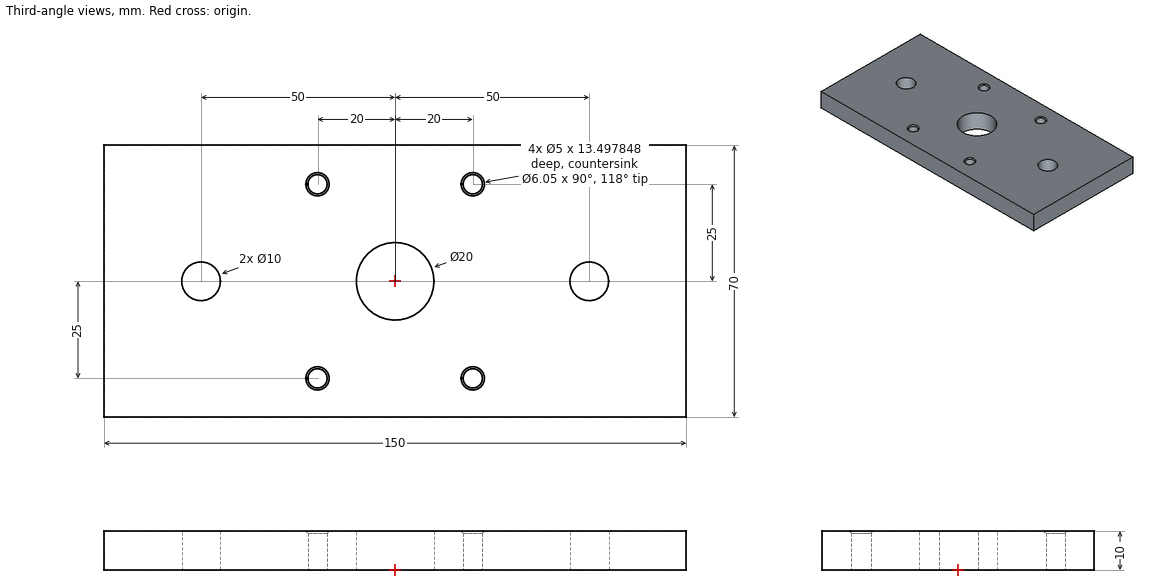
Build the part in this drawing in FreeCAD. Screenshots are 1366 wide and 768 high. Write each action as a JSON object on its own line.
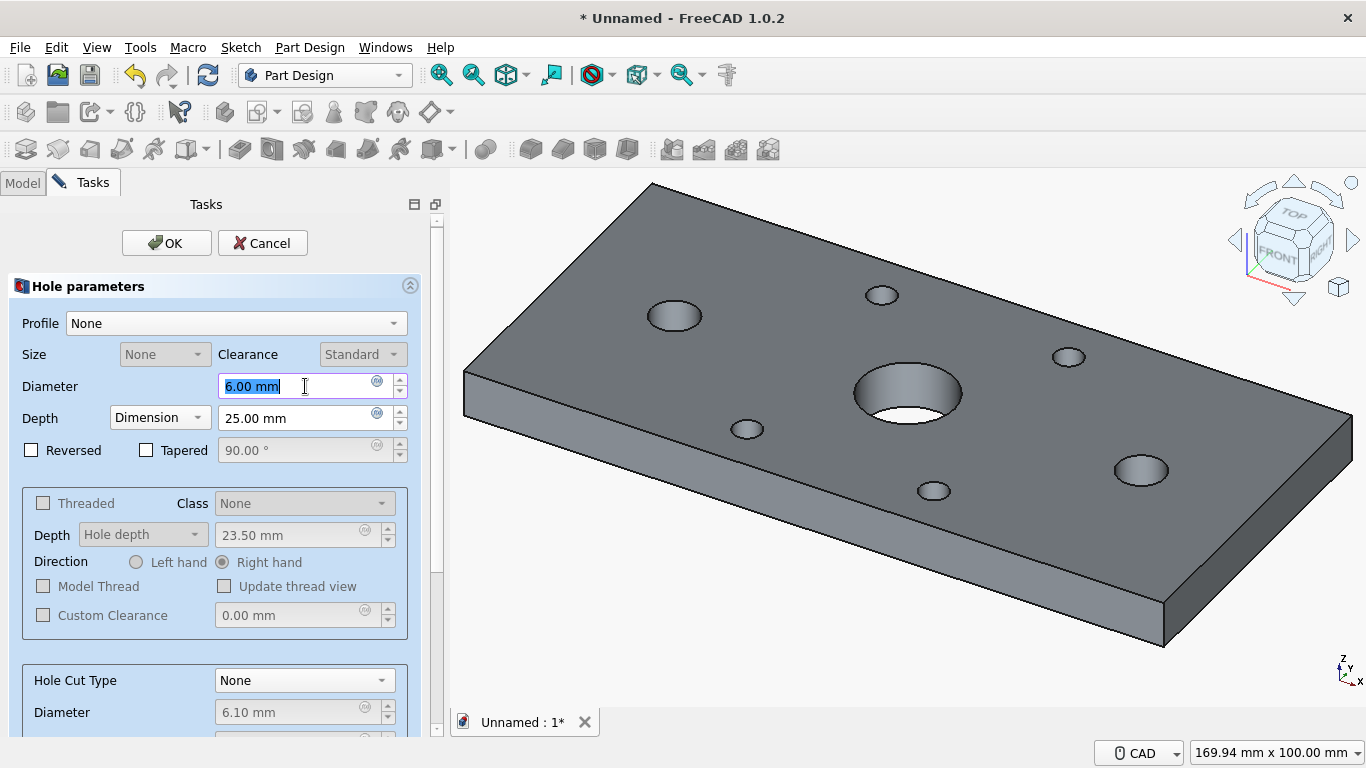
{"action": "type", "text": "5"}
{"action": "key", "text": "Tab"}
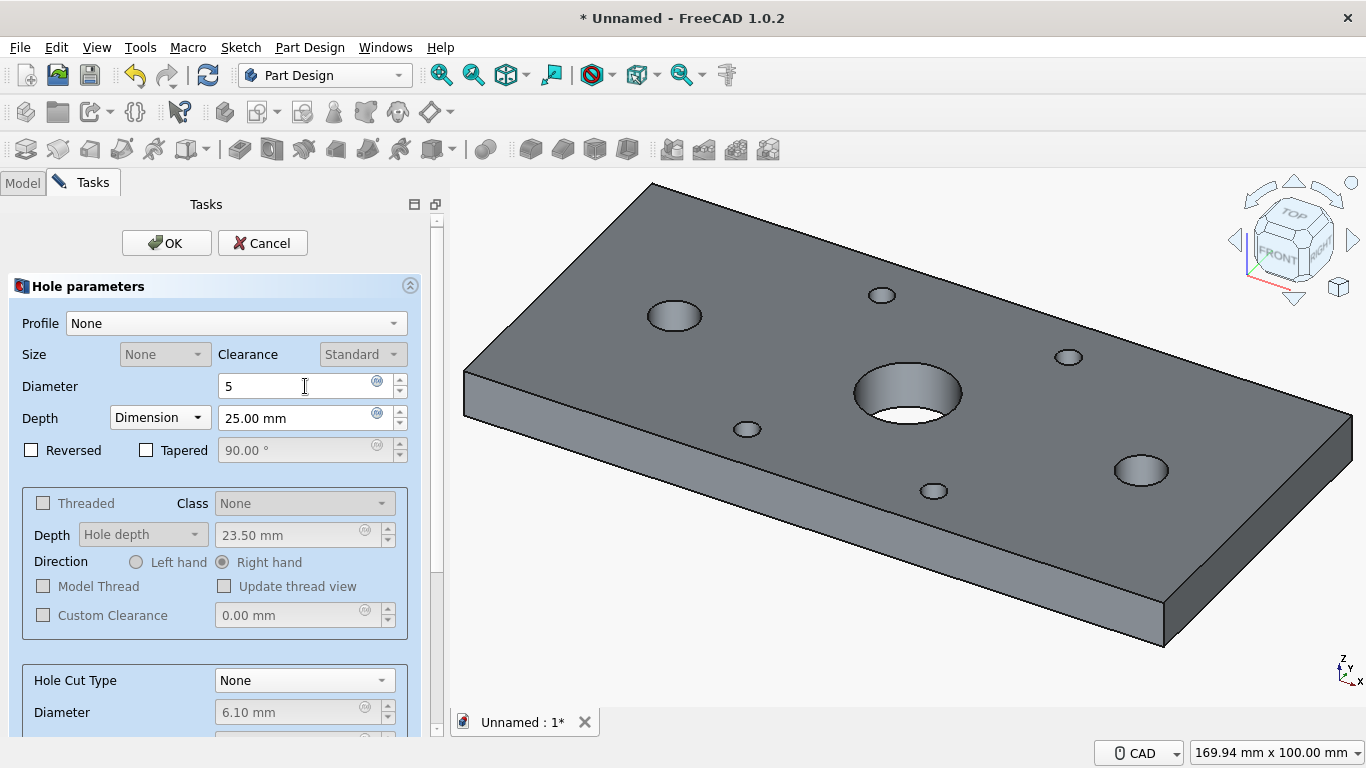
{"action": "triple_click", "coordinate": [305, 418]}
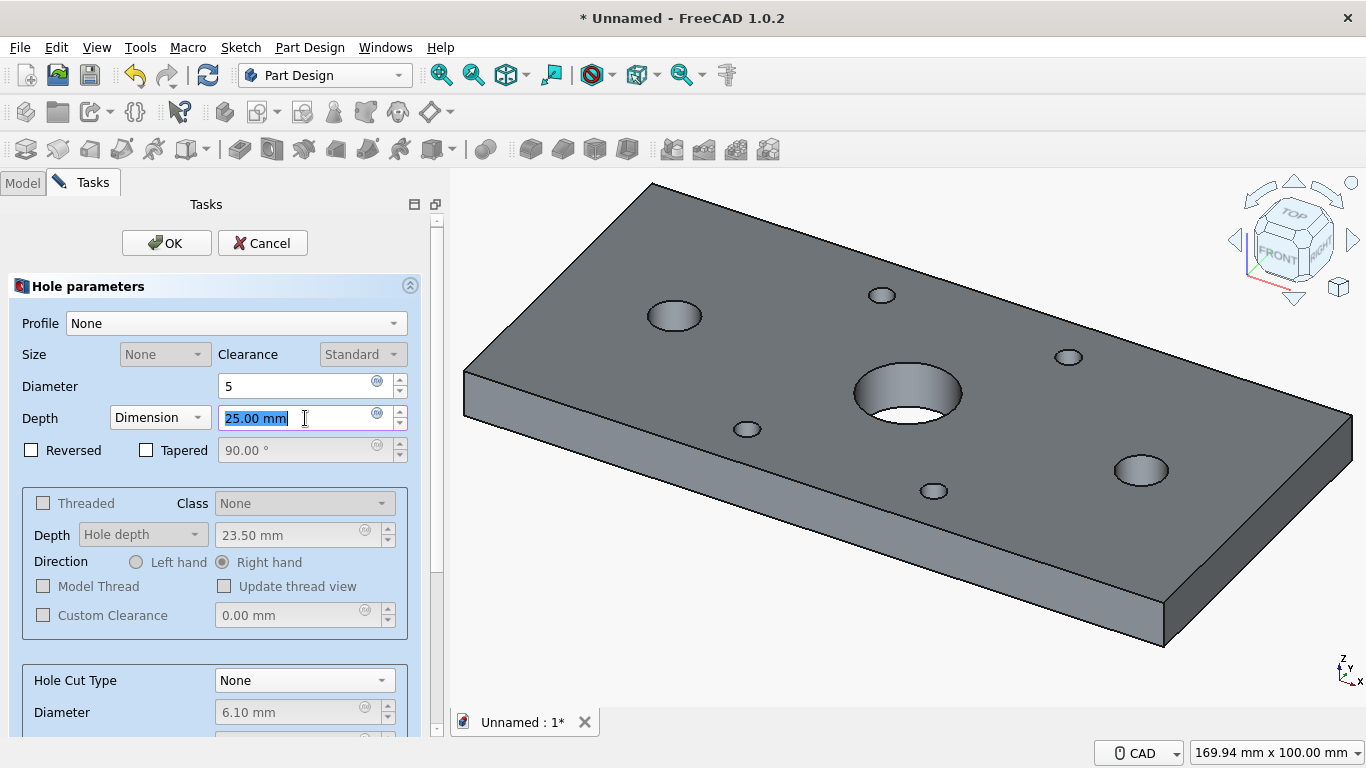
{"action": "type", "text": "13.497848"}
{"action": "key", "text": "Tab"}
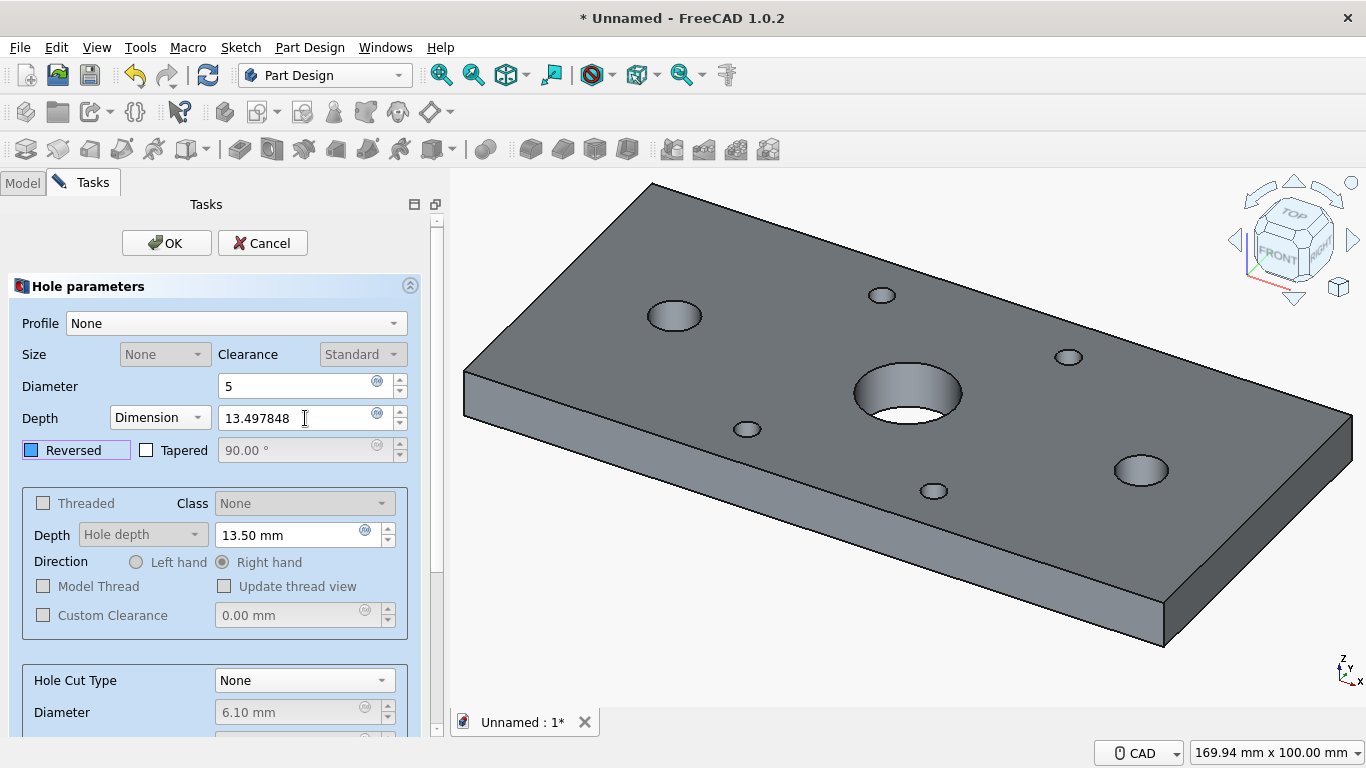
{"action": "left_click", "coordinate": [306, 680]}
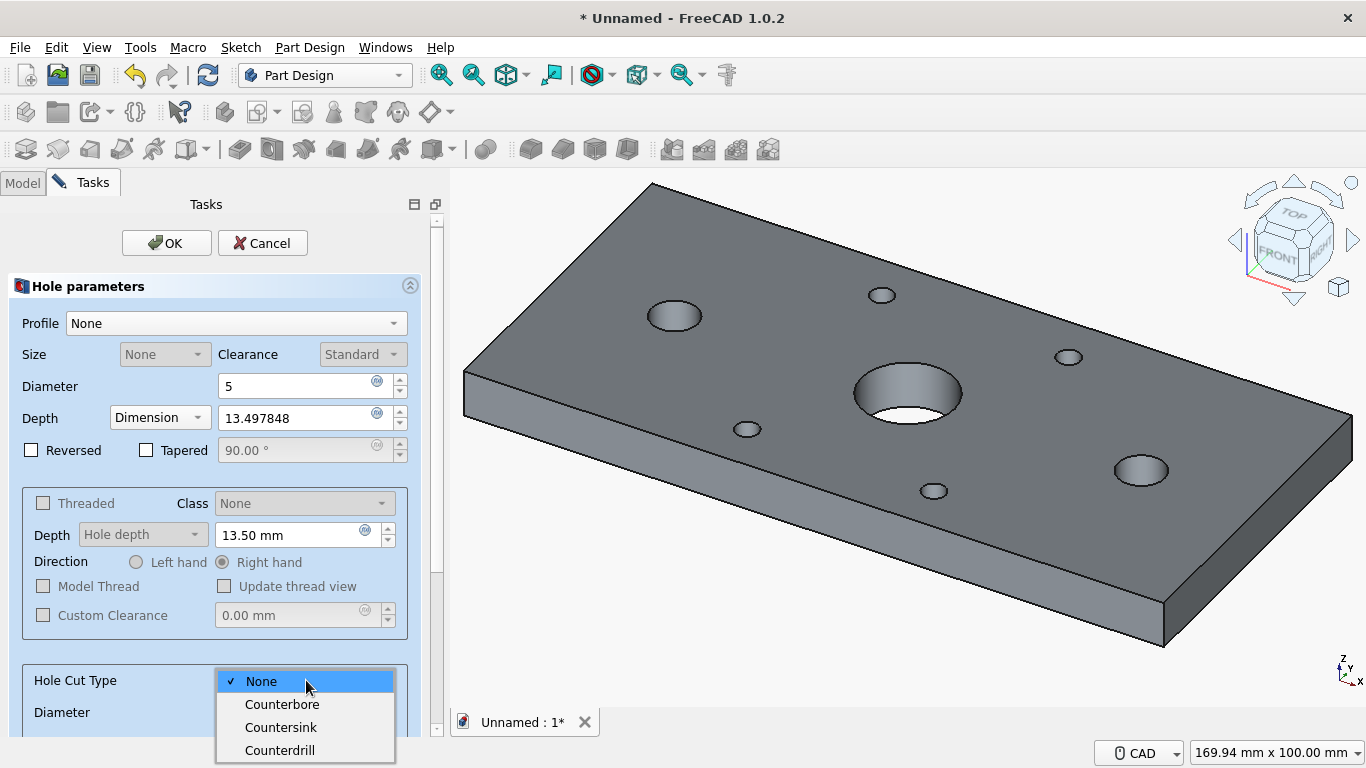
{"action": "left_click", "coordinate": [304, 728]}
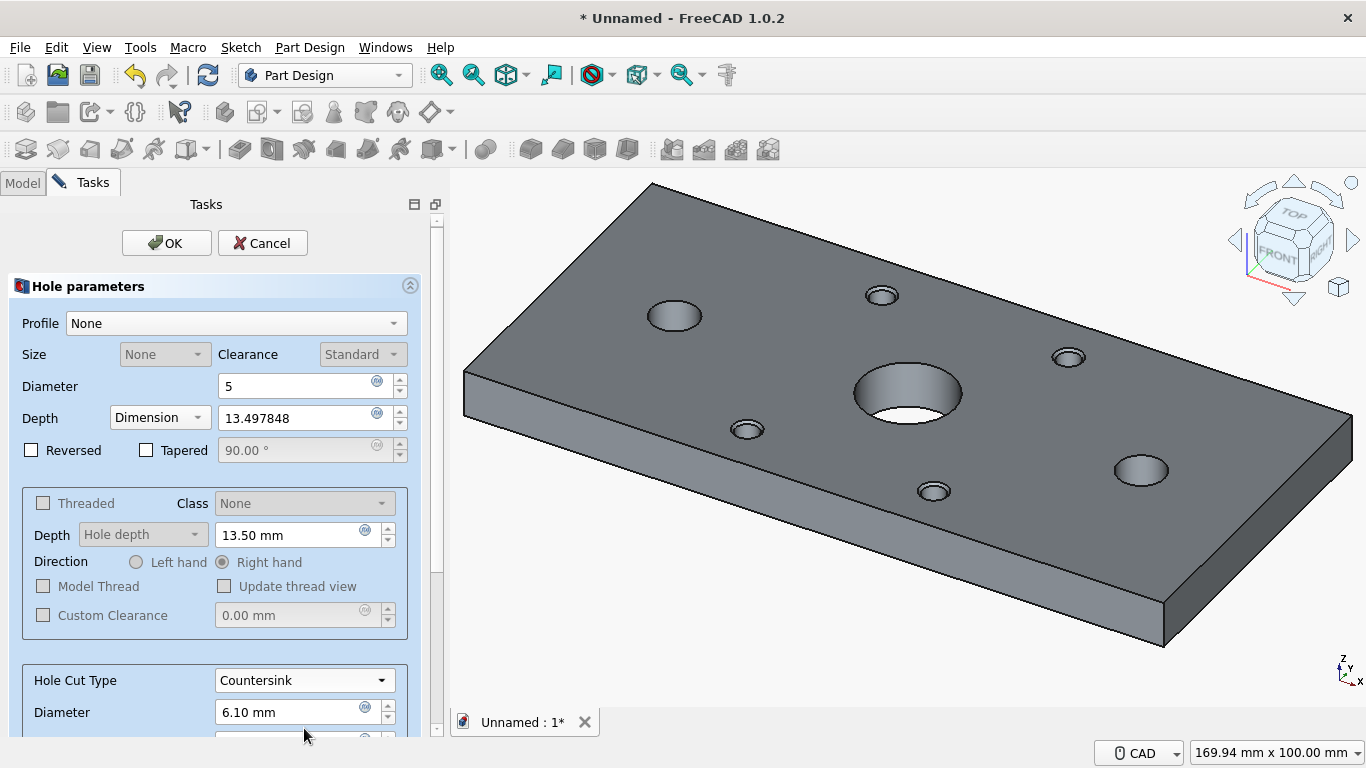
{"action": "triple_click", "coordinate": [298, 712]}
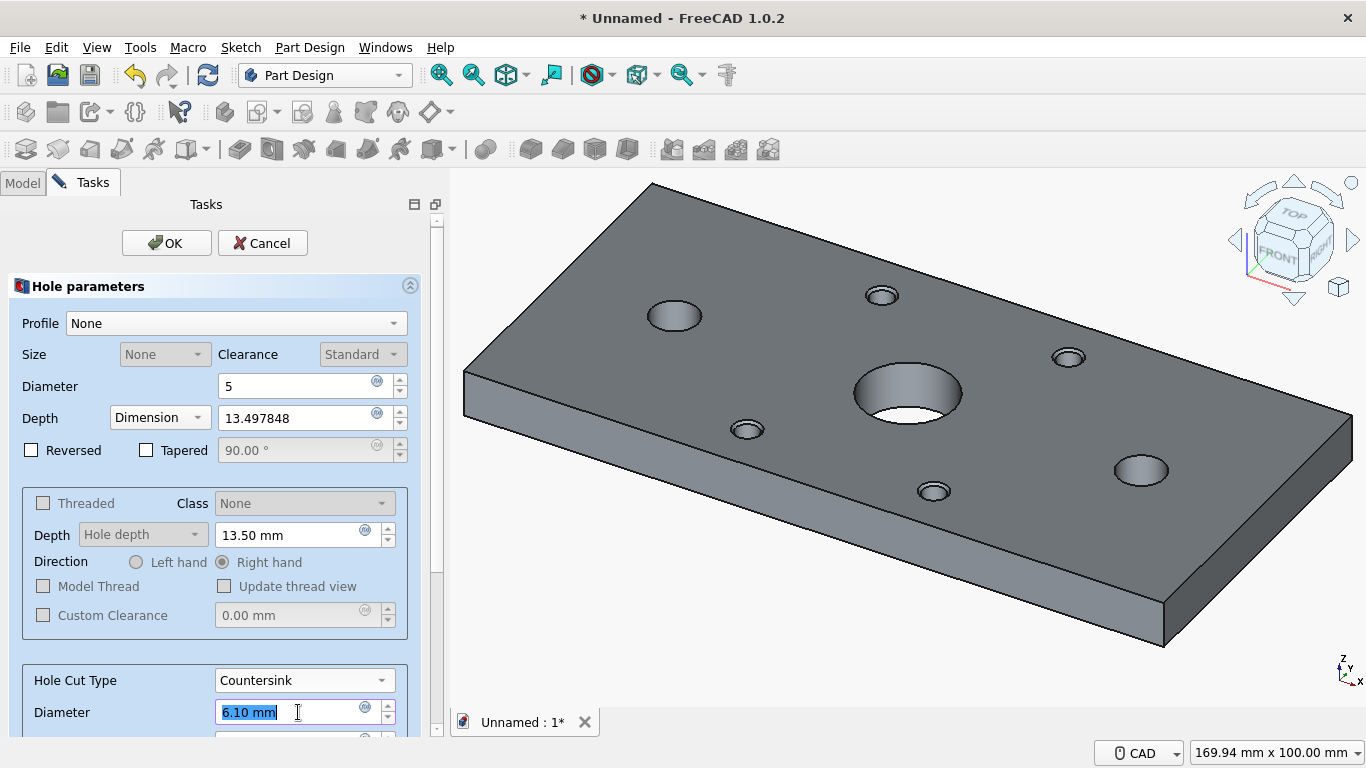
{"action": "type", "text": "6.05"}
{"action": "key", "text": "Tab"}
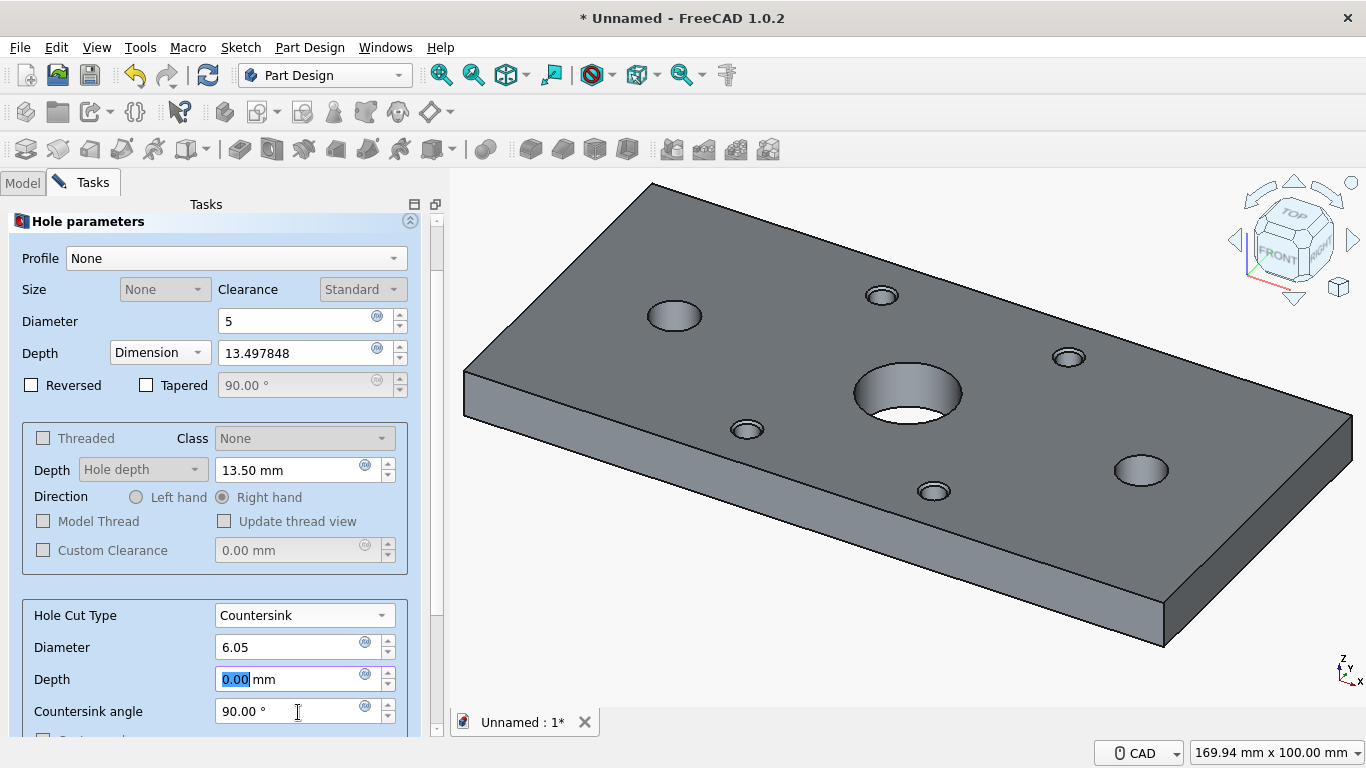
{"action": "scroll", "coordinate": [437, 475], "scroll_direction": "up", "scroll_amount": 2}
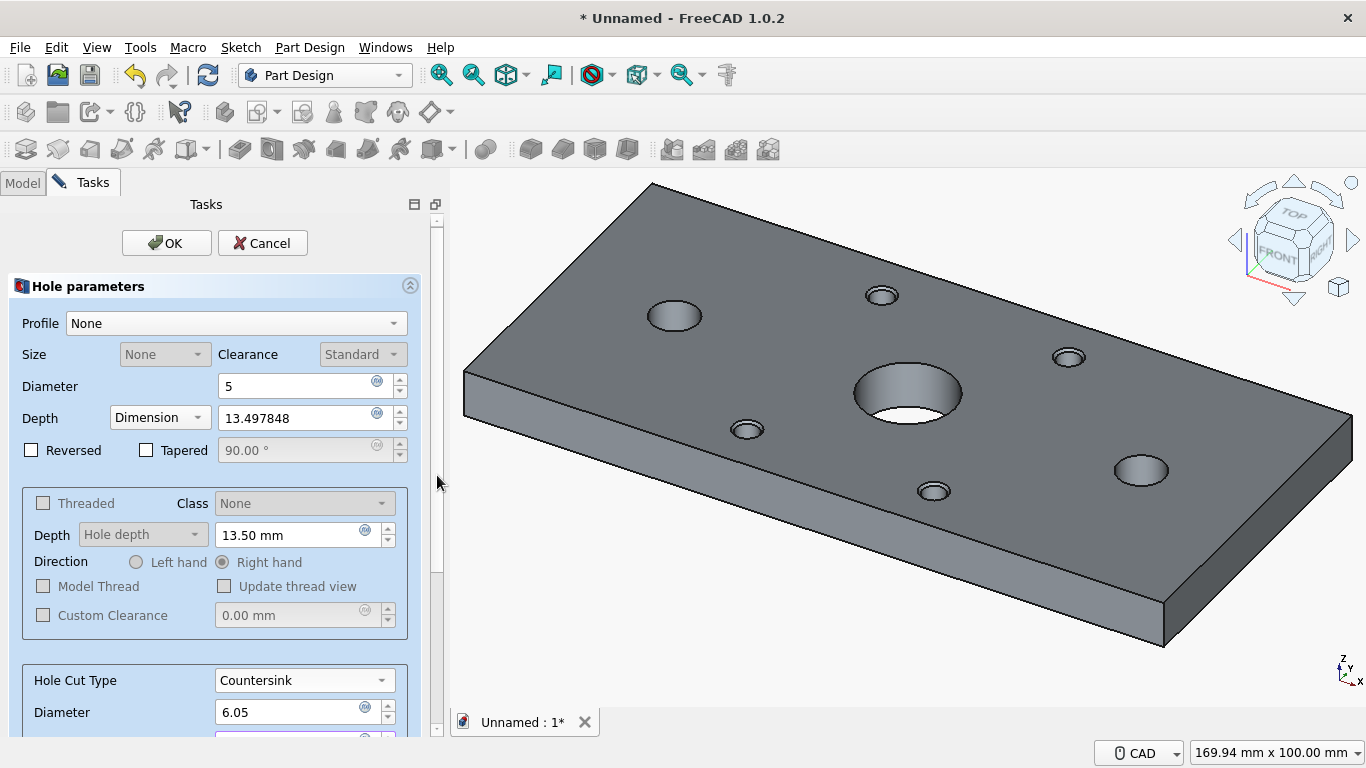
{"action": "left_click", "coordinate": [167, 243]}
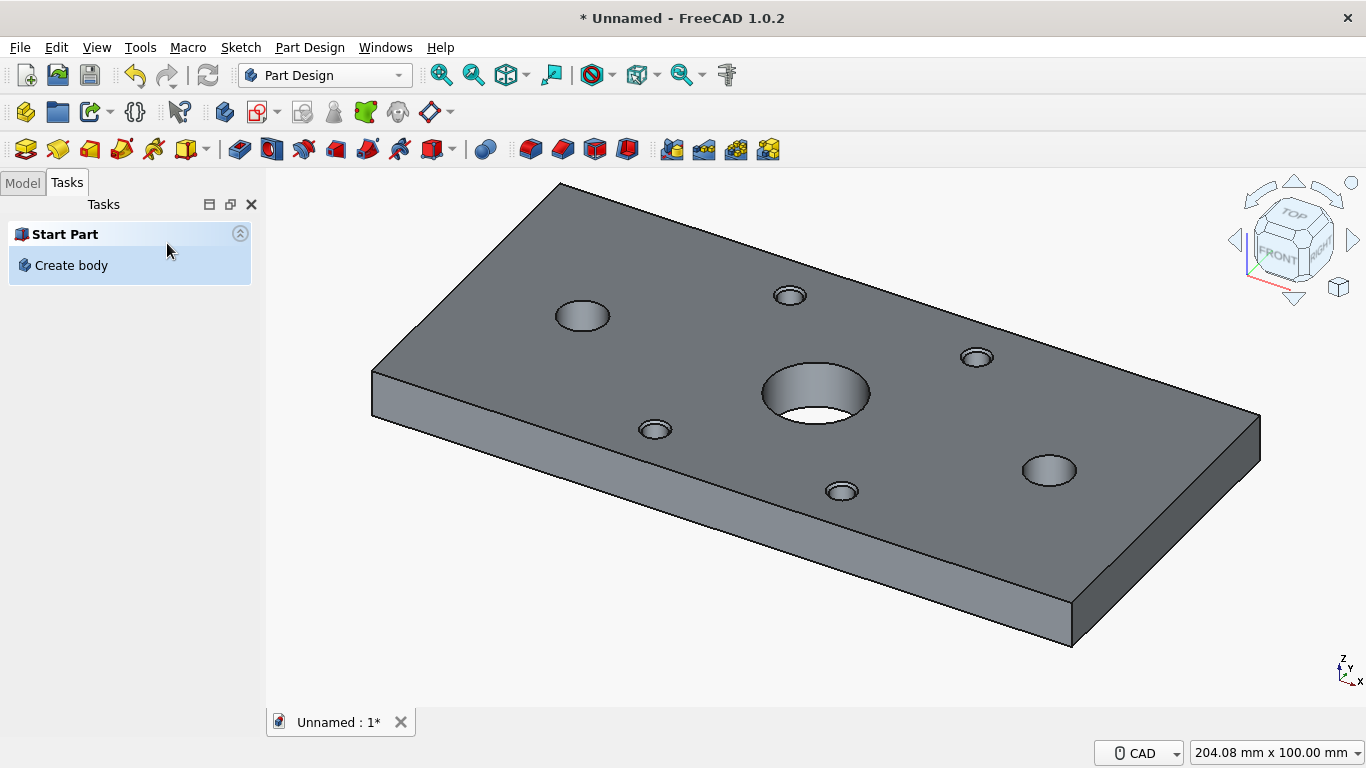
{"action": "key", "text": "0"}